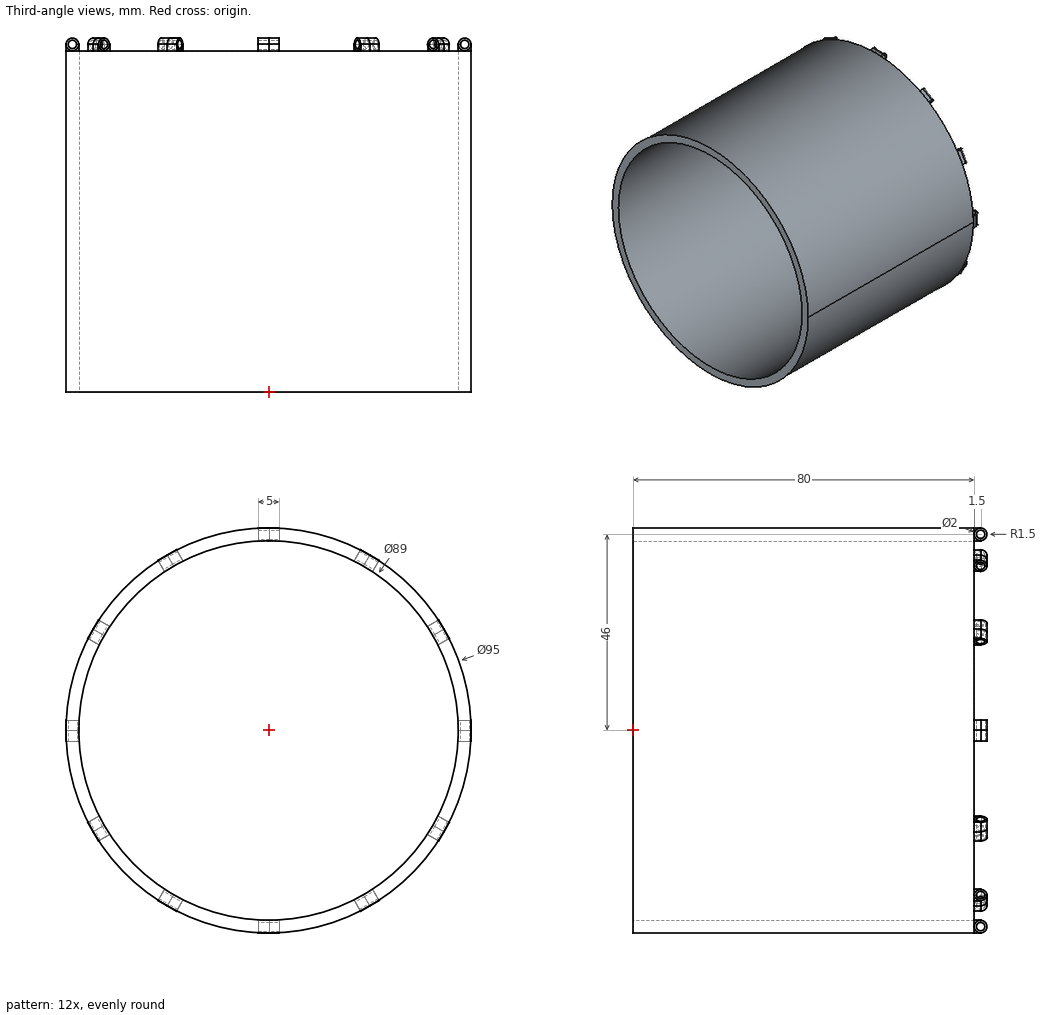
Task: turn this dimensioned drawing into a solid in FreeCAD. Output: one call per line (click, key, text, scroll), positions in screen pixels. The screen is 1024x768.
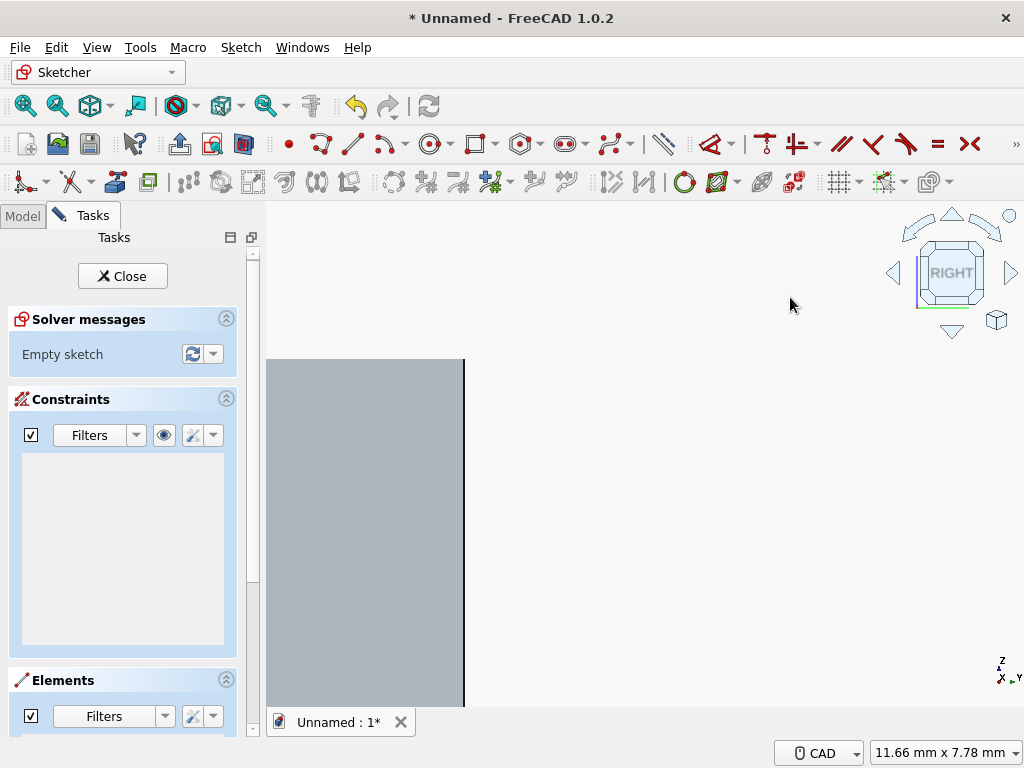
scroll(532, 463, up, 2)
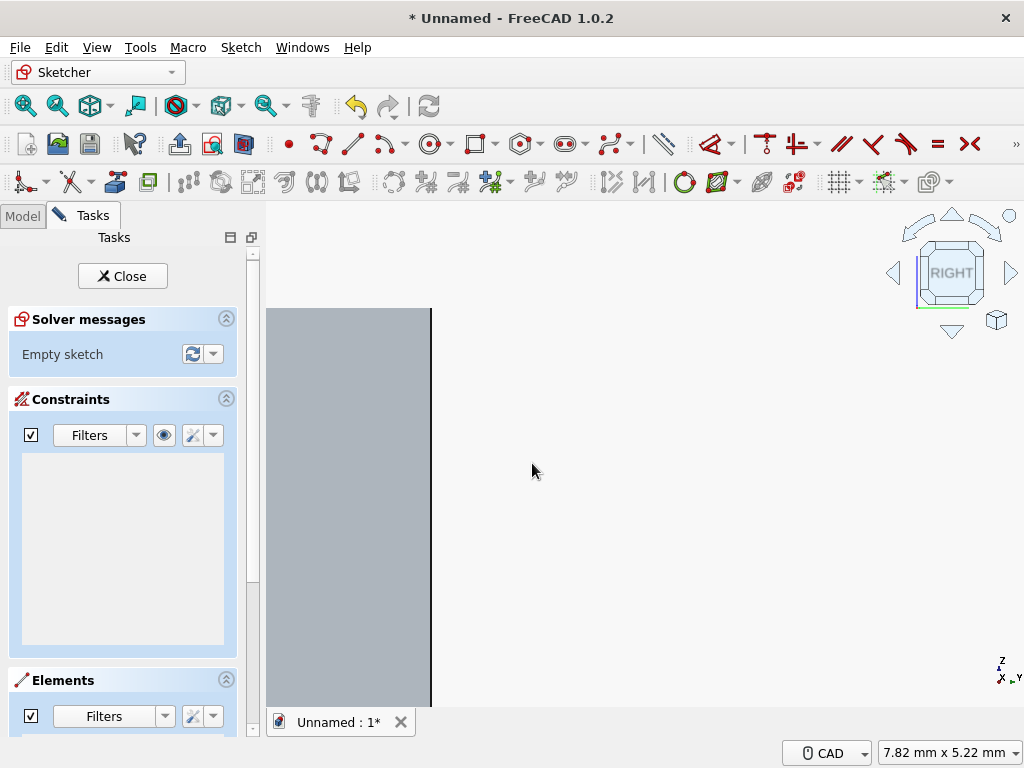
click(322, 144)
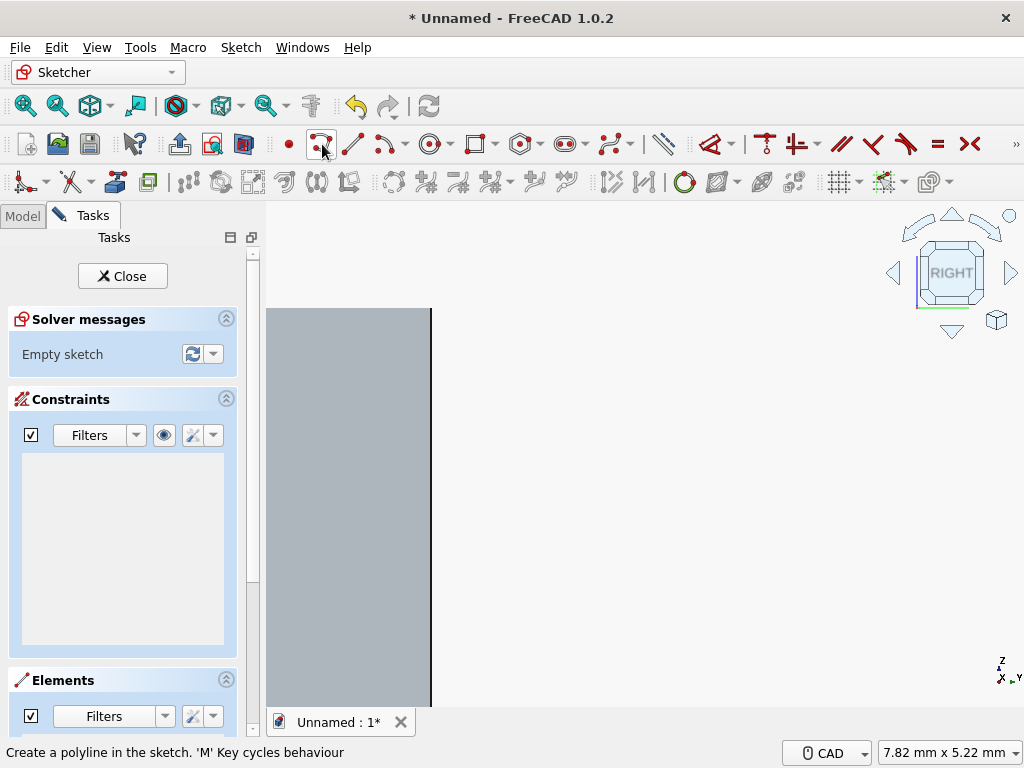
click(576, 308)
click(431, 308)
click(431, 599)
click(576, 599)
right_click(576, 599)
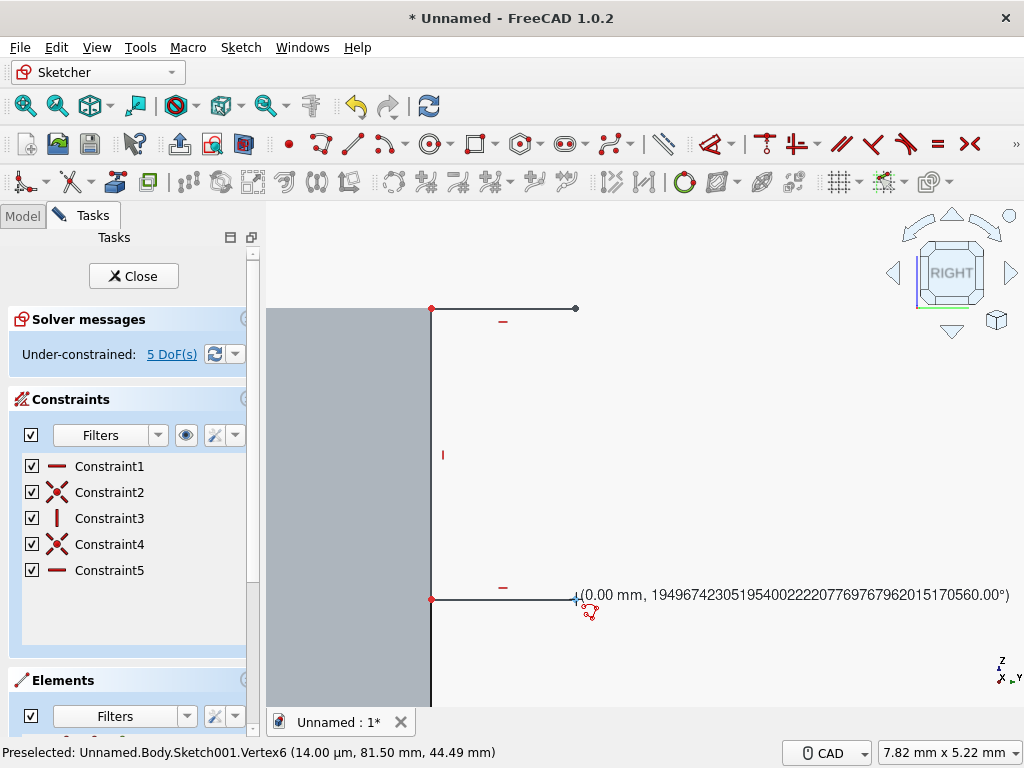
key(g)
key(3)
key(a)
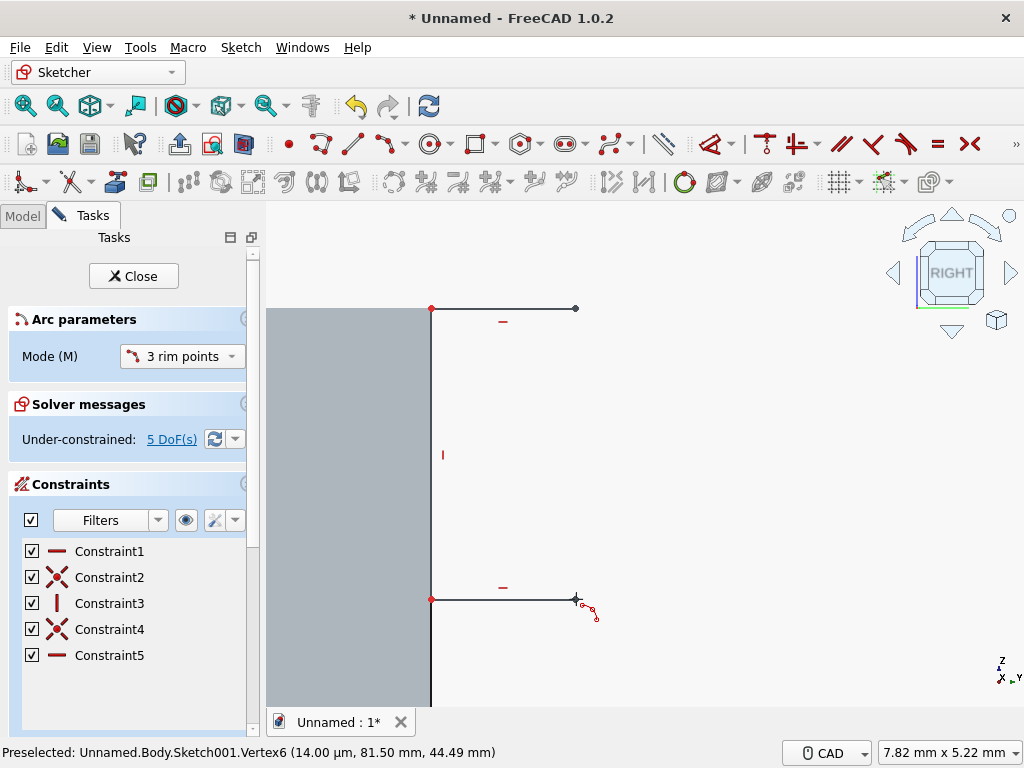
click(576, 600)
click(576, 309)
click(722, 454)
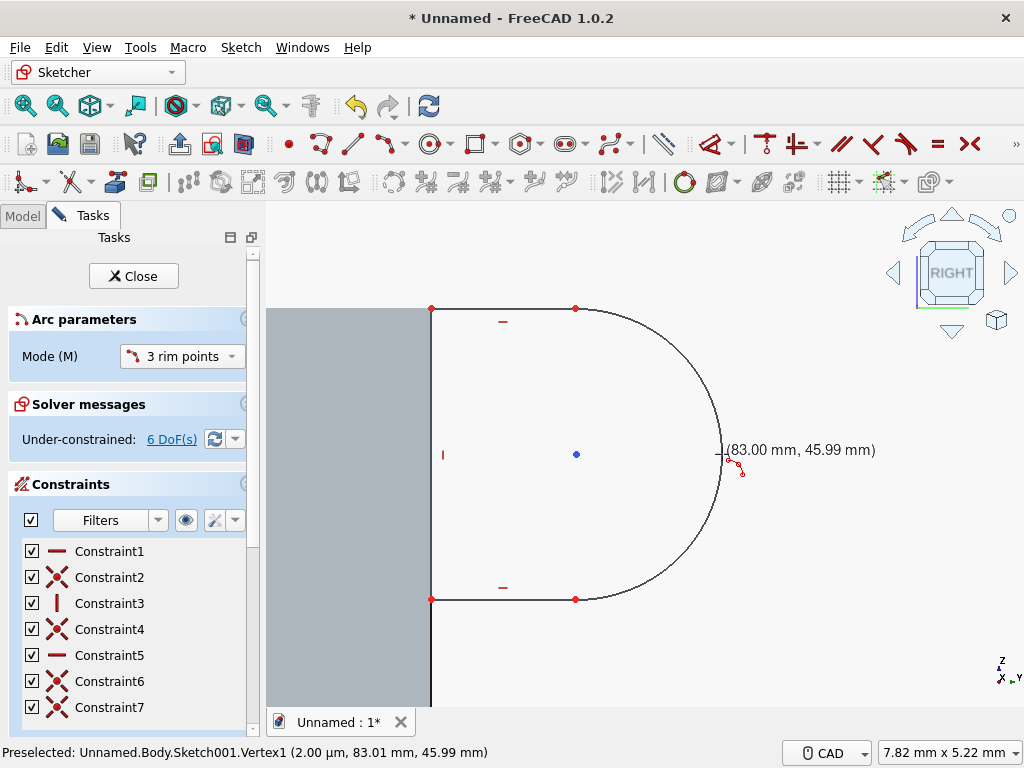
key(g)
key(c)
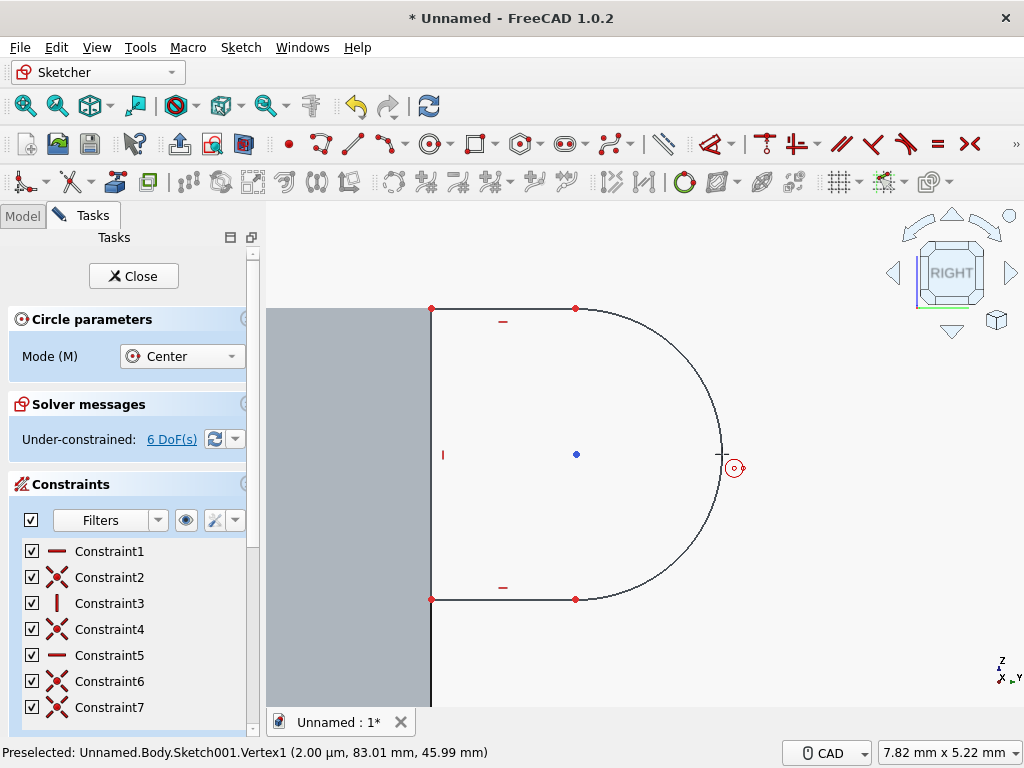
click(576, 454)
click(645, 385)
key(Escape)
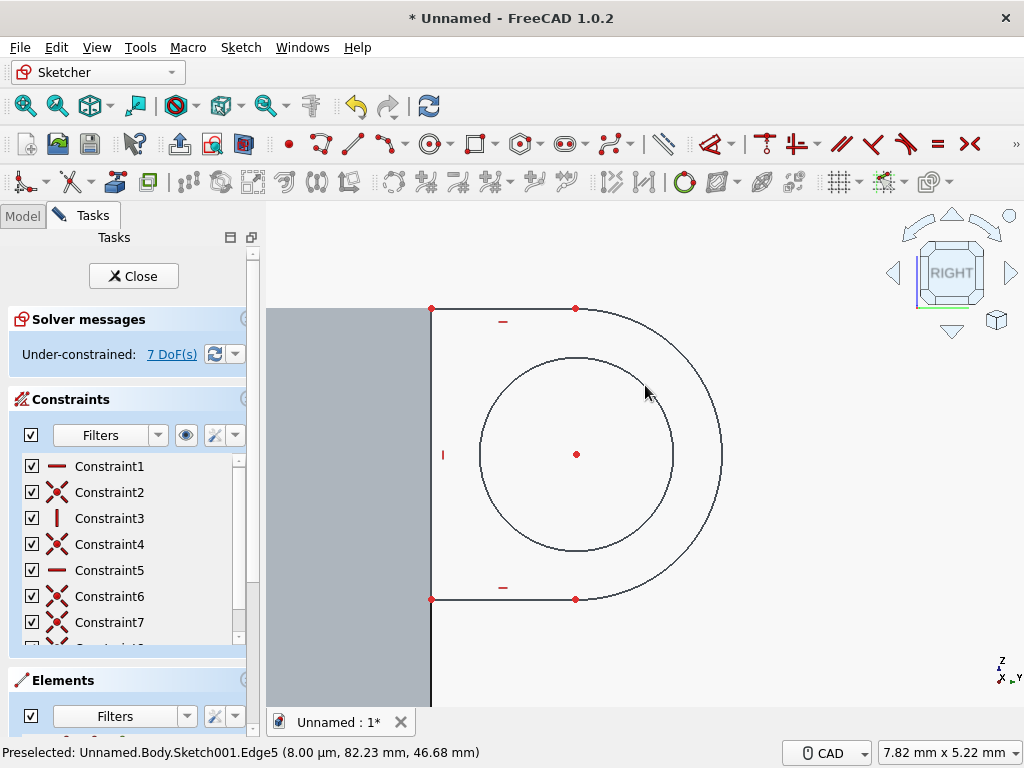
click(532, 309)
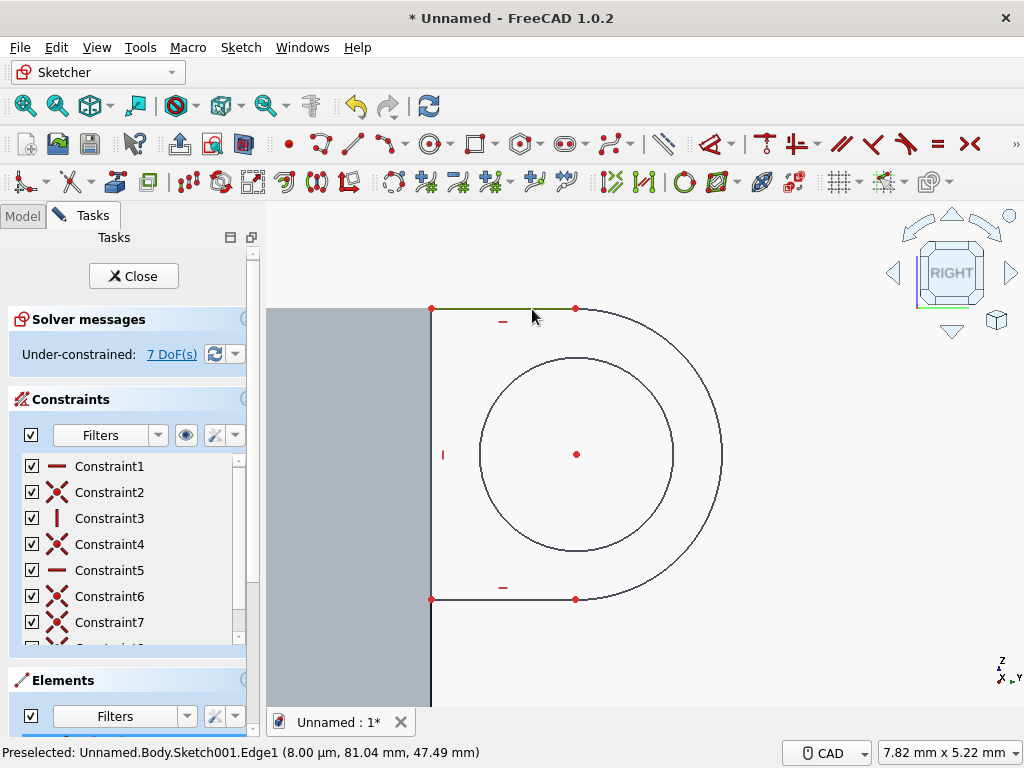
click(694, 540)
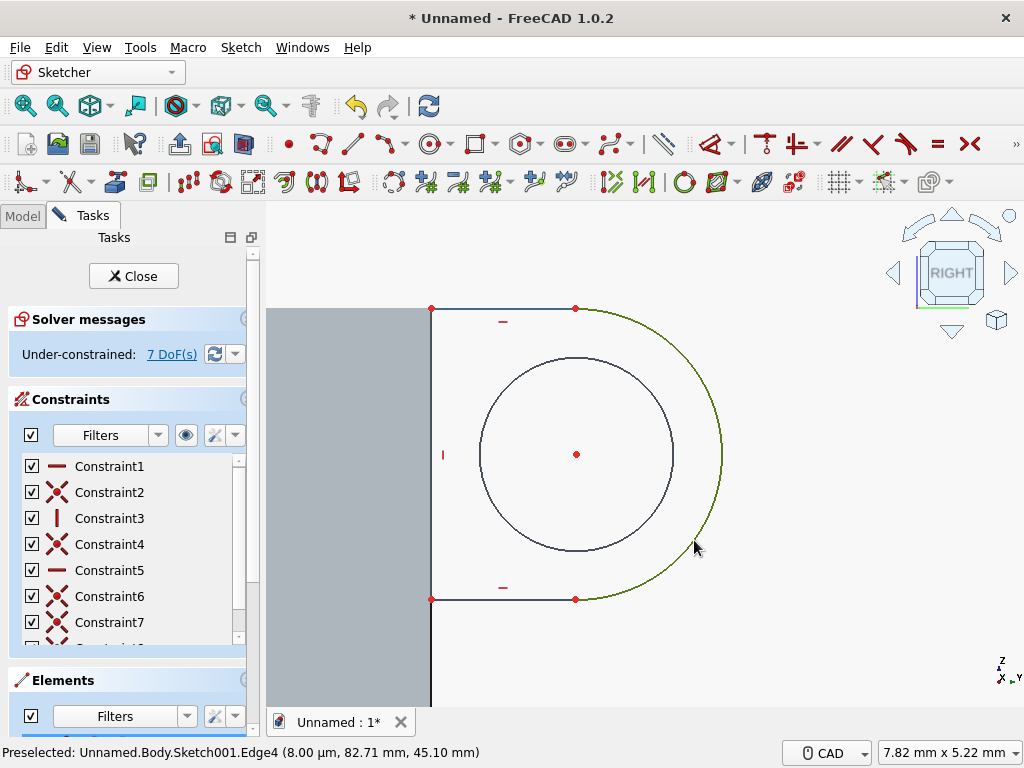
click(906, 144)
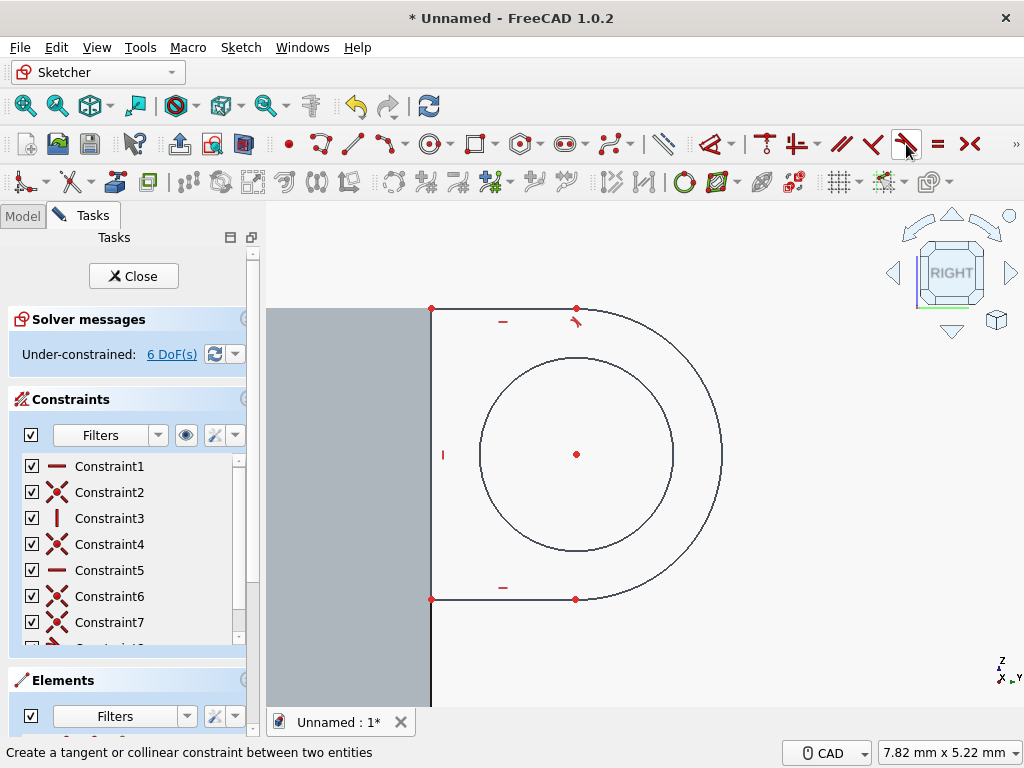
click(474, 600)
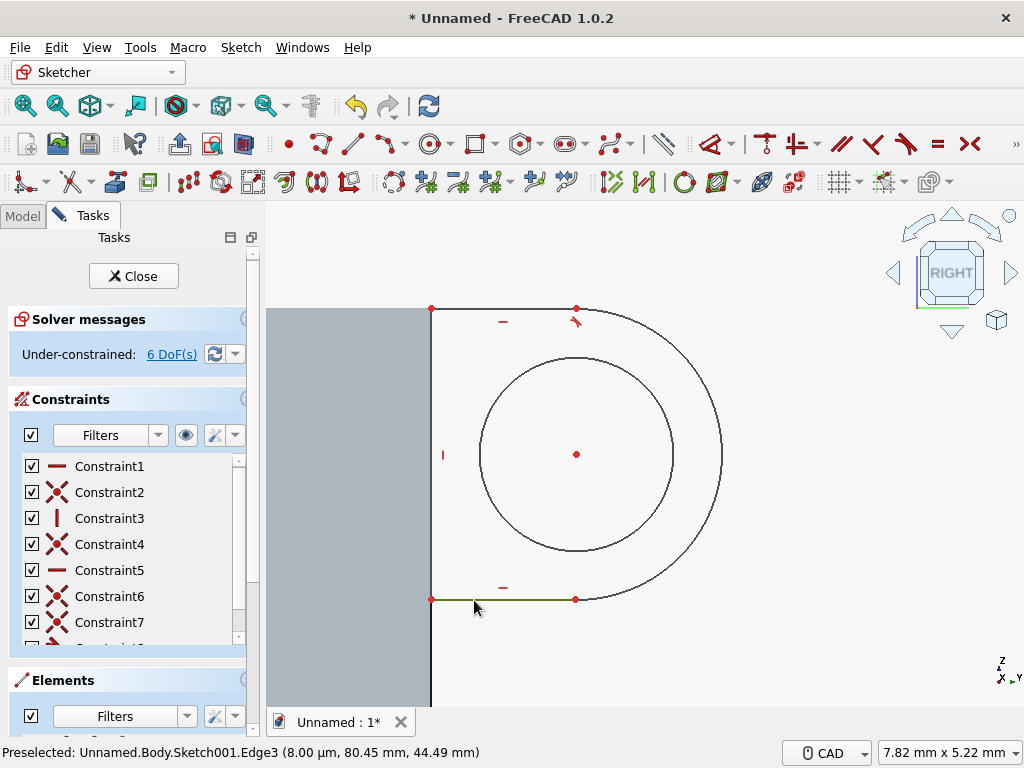
click(694, 540)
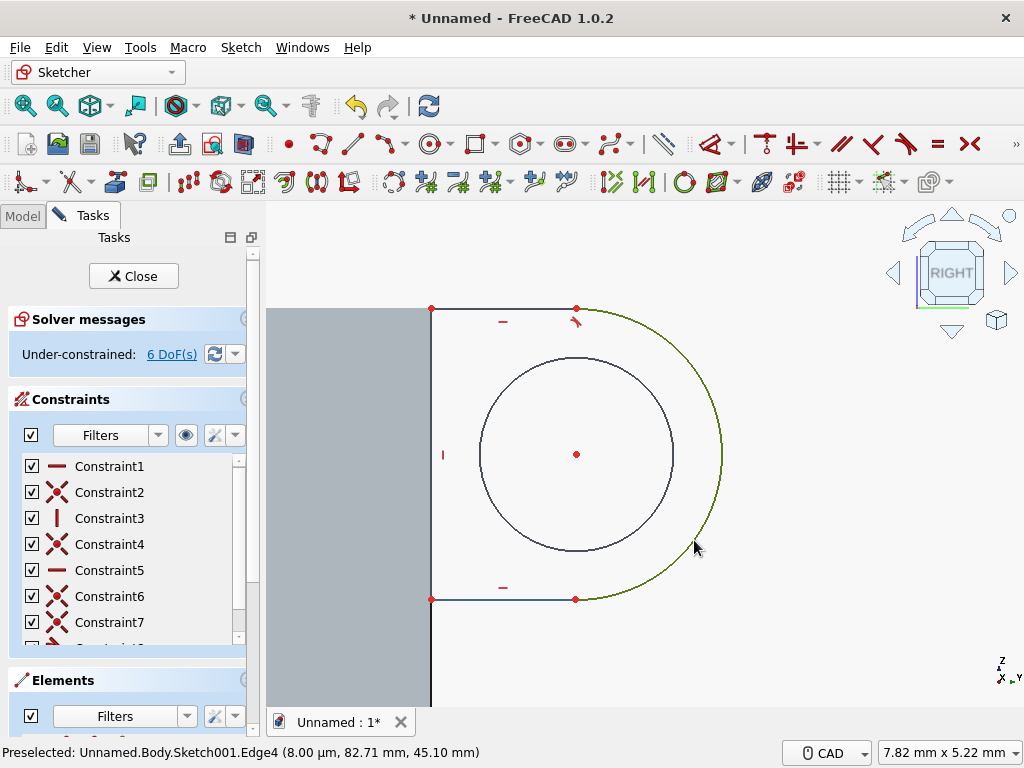
click(906, 144)